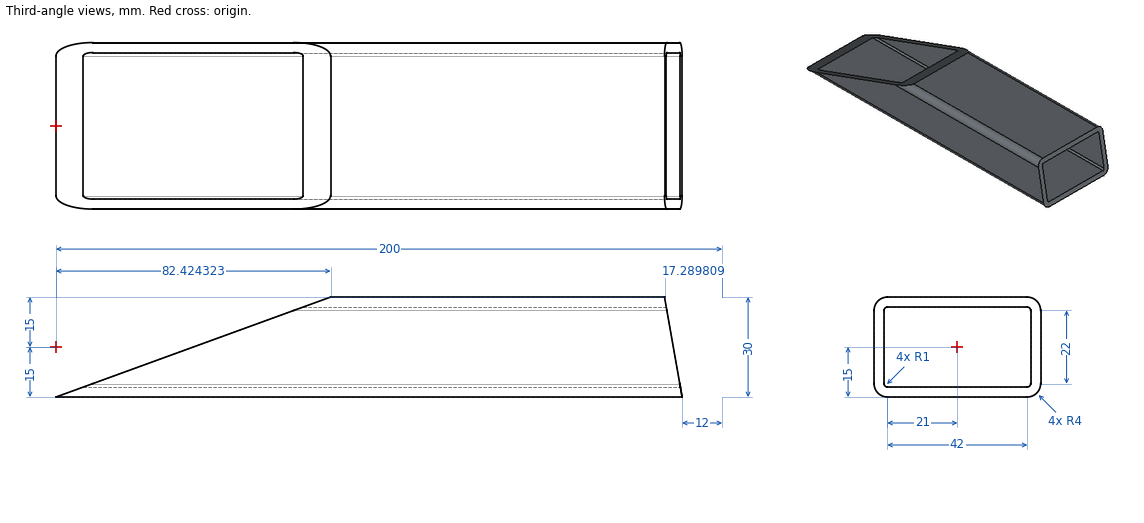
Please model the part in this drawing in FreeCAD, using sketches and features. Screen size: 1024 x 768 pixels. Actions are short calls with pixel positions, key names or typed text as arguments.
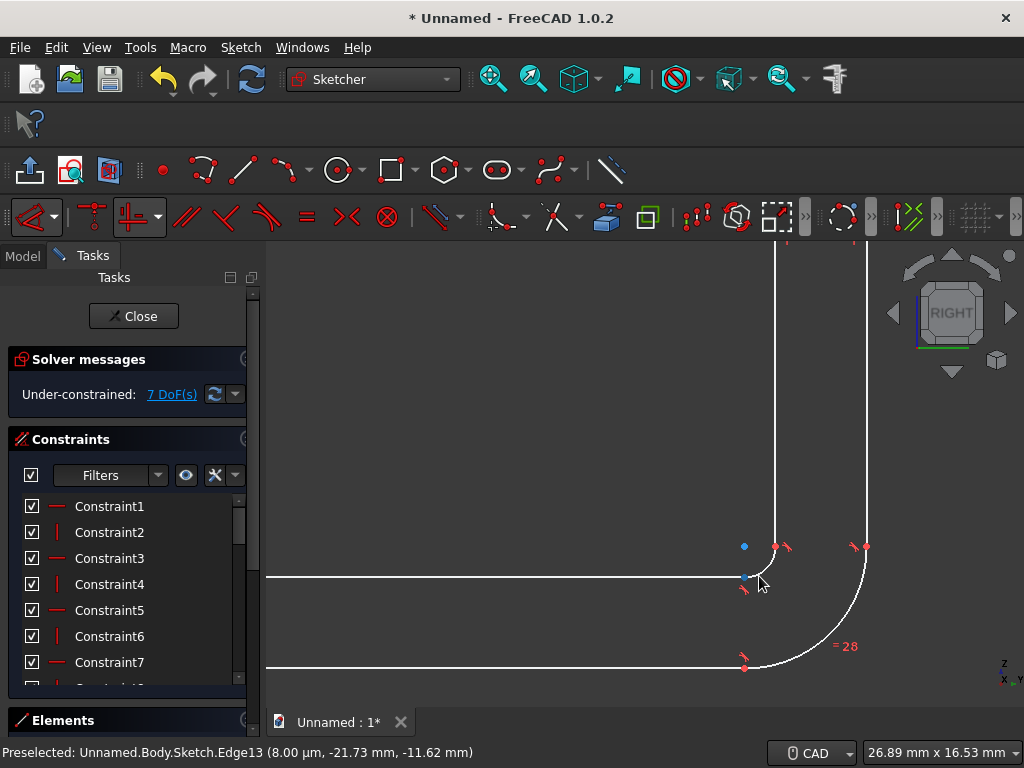
click(759, 574)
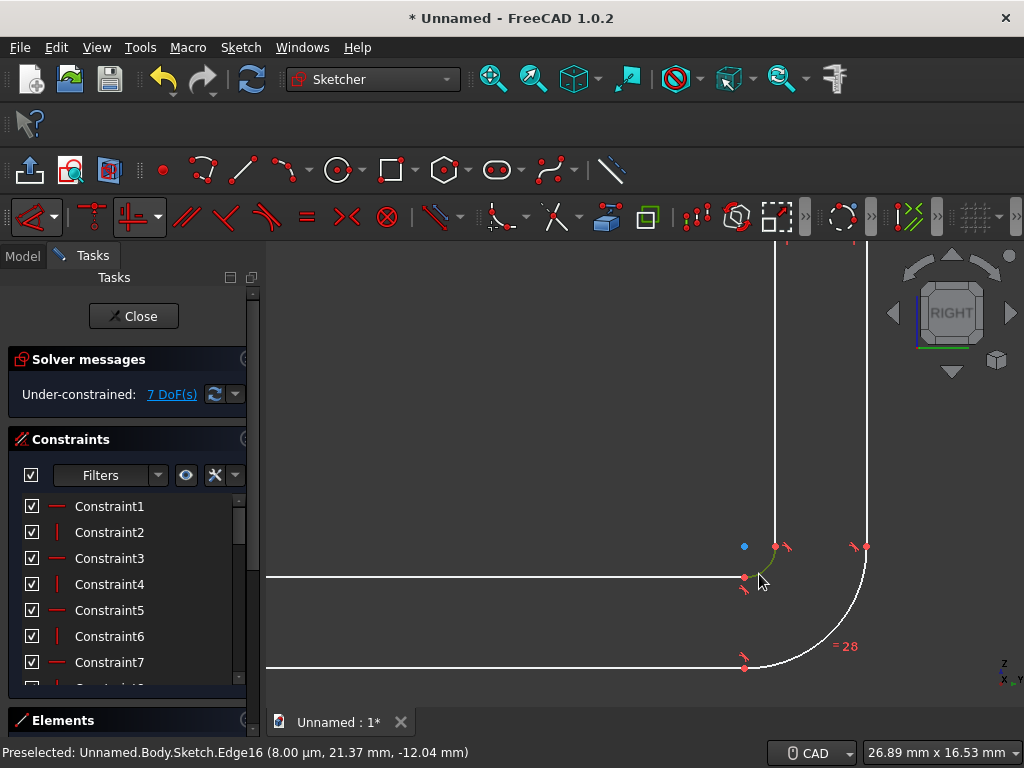
click(308, 218)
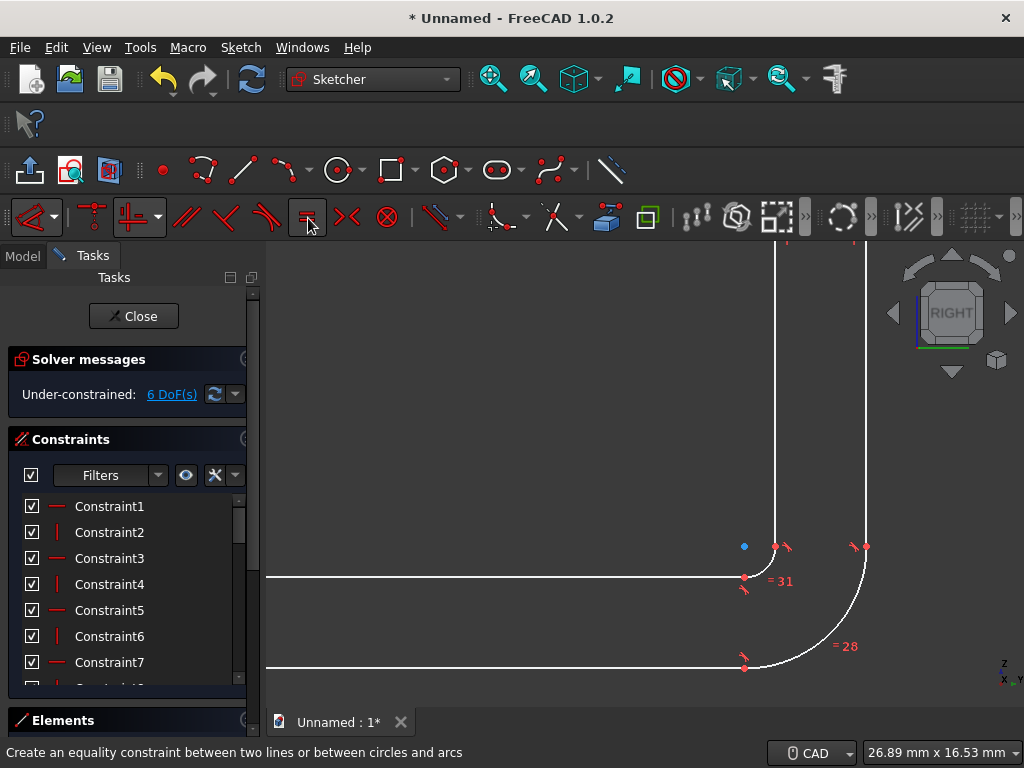
click(30, 218)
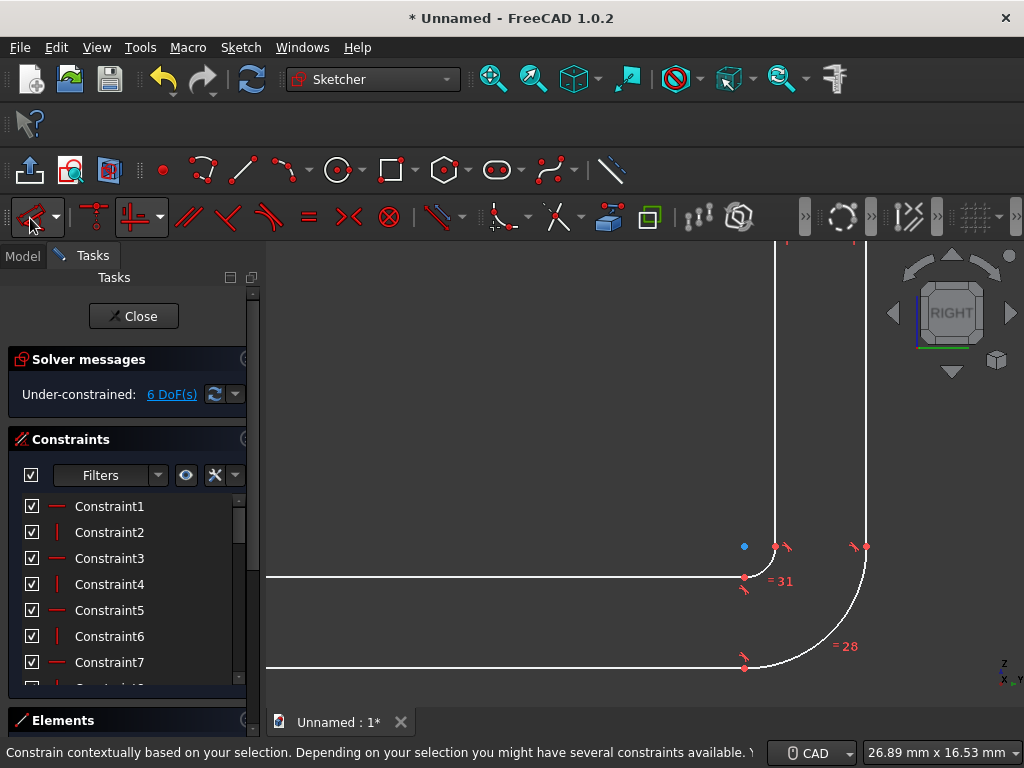
click(800, 655)
click(608, 617)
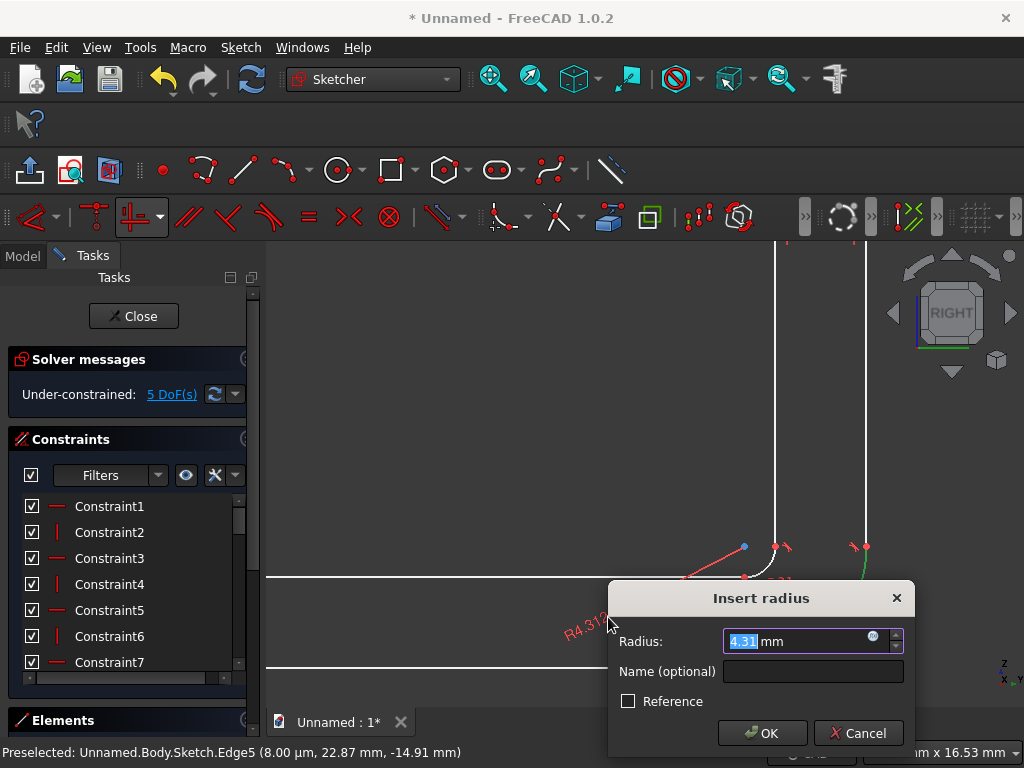
text(4)
key(Return)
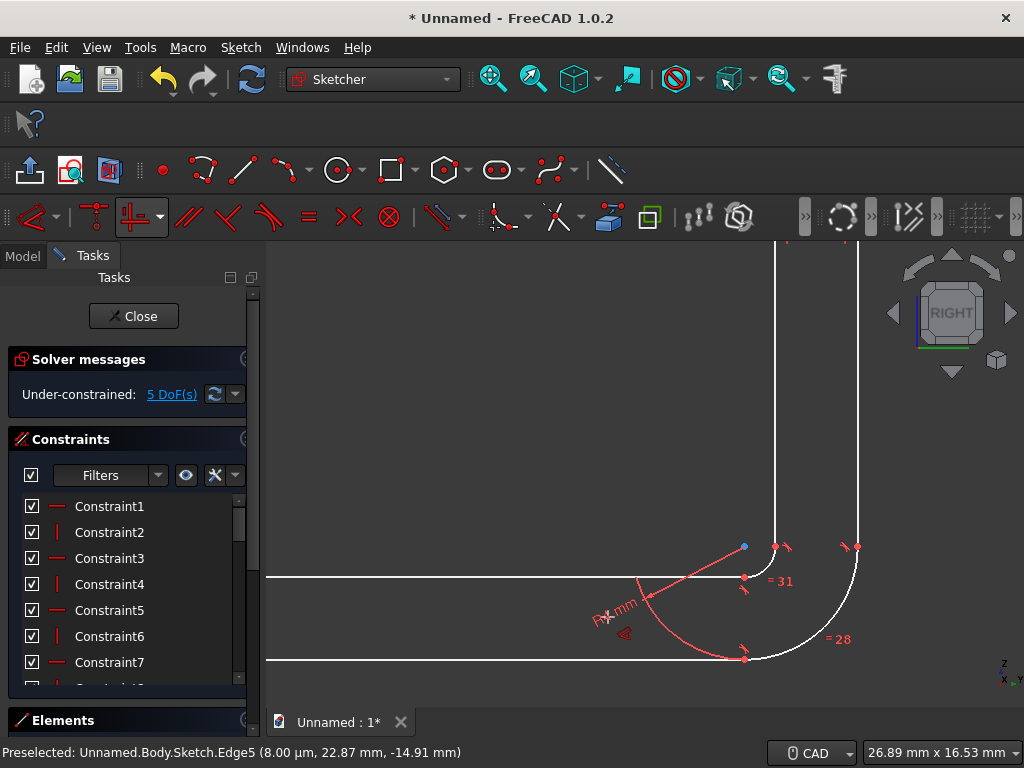
scroll(759, 576, down, 6)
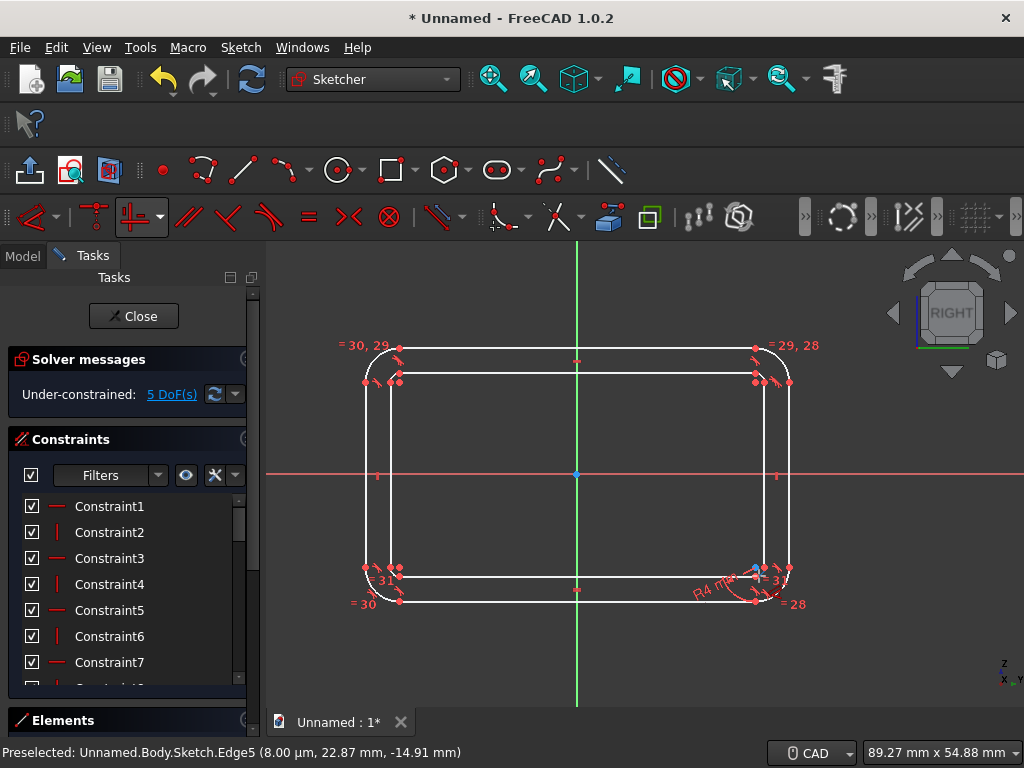
scroll(392, 572, up, 8)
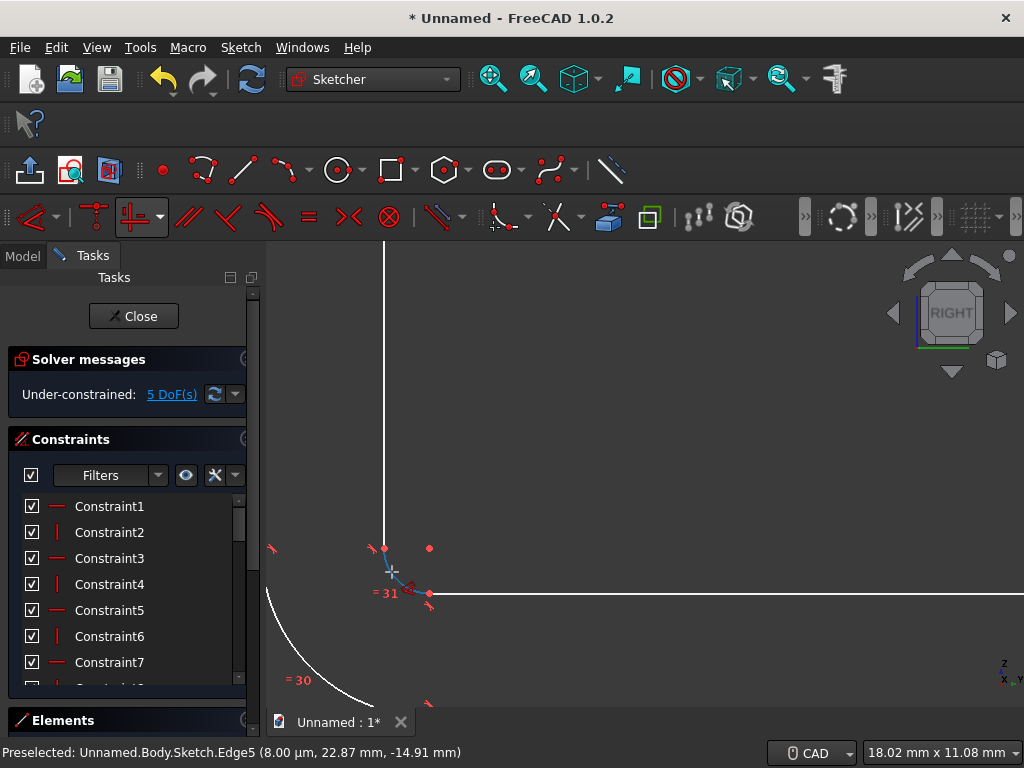
click(389, 569)
click(361, 584)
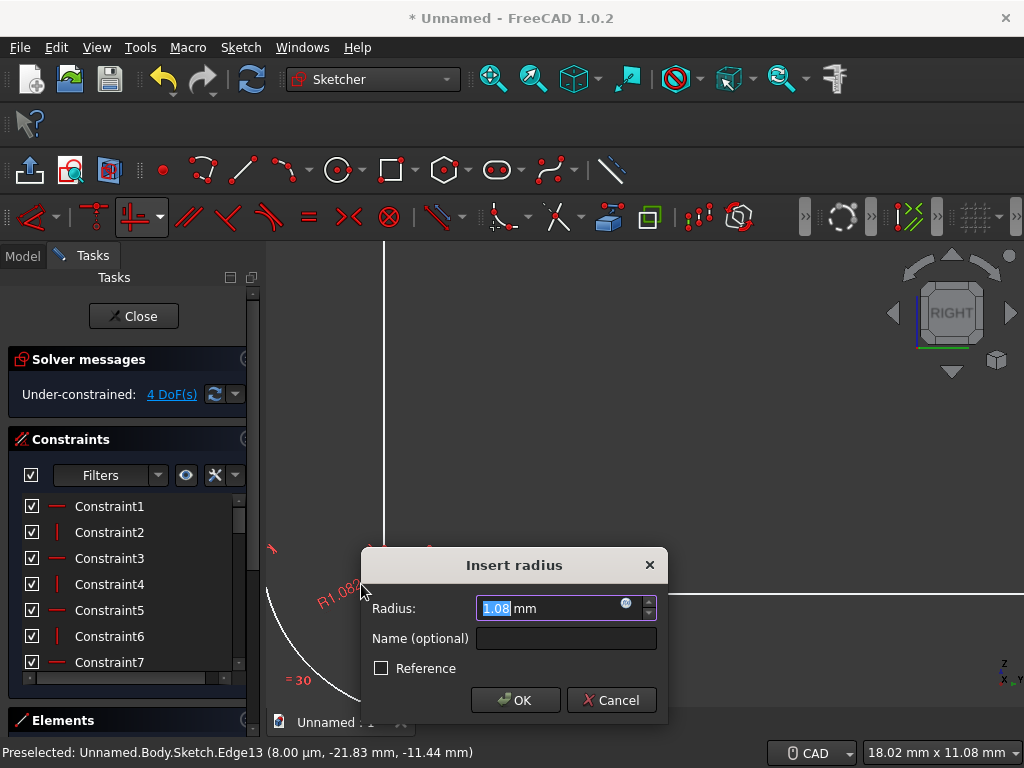
text(1)
key(Return)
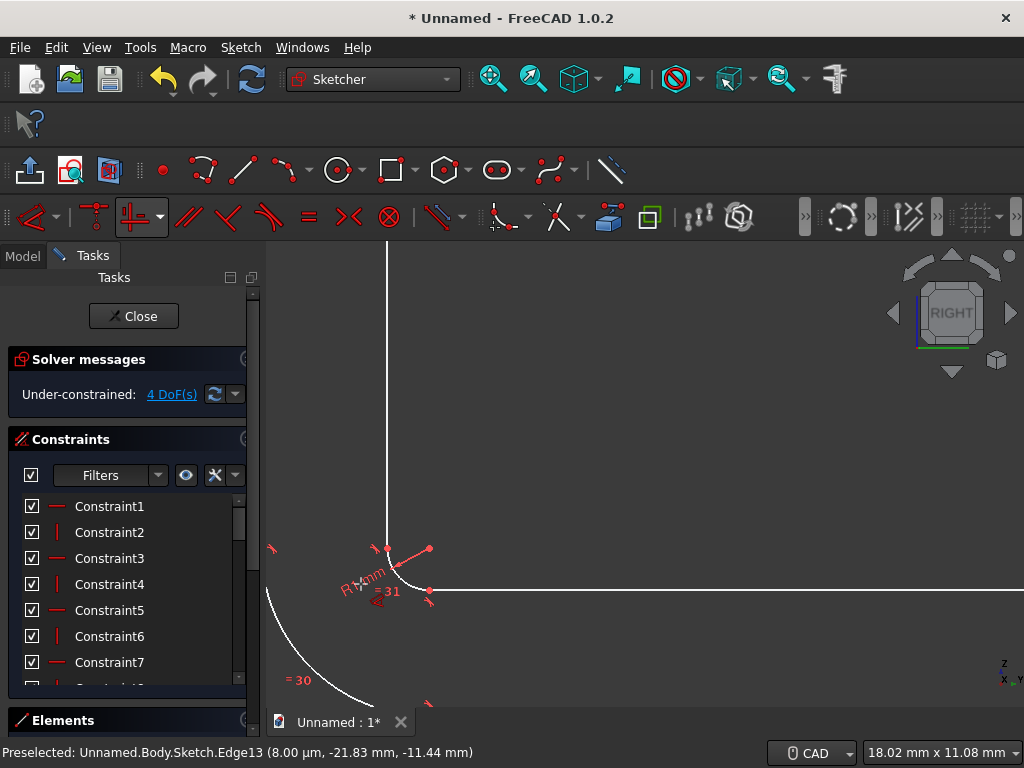
scroll(392, 572, down, 8)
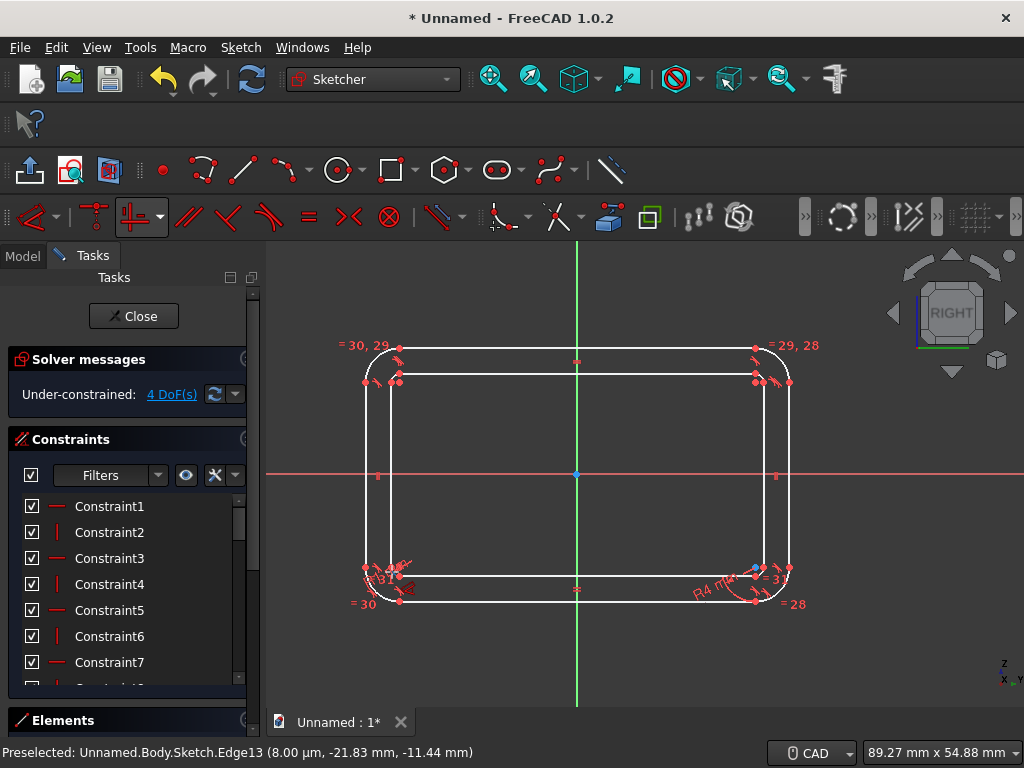
click(506, 602)
click(496, 636)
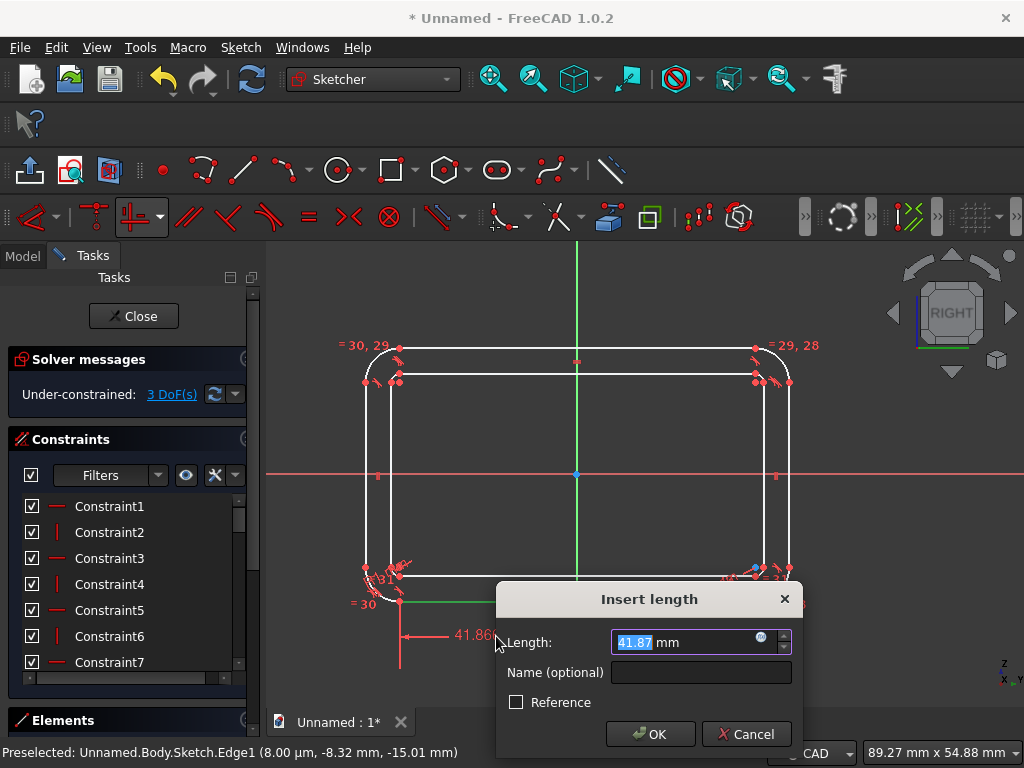
text(42)
key(Return)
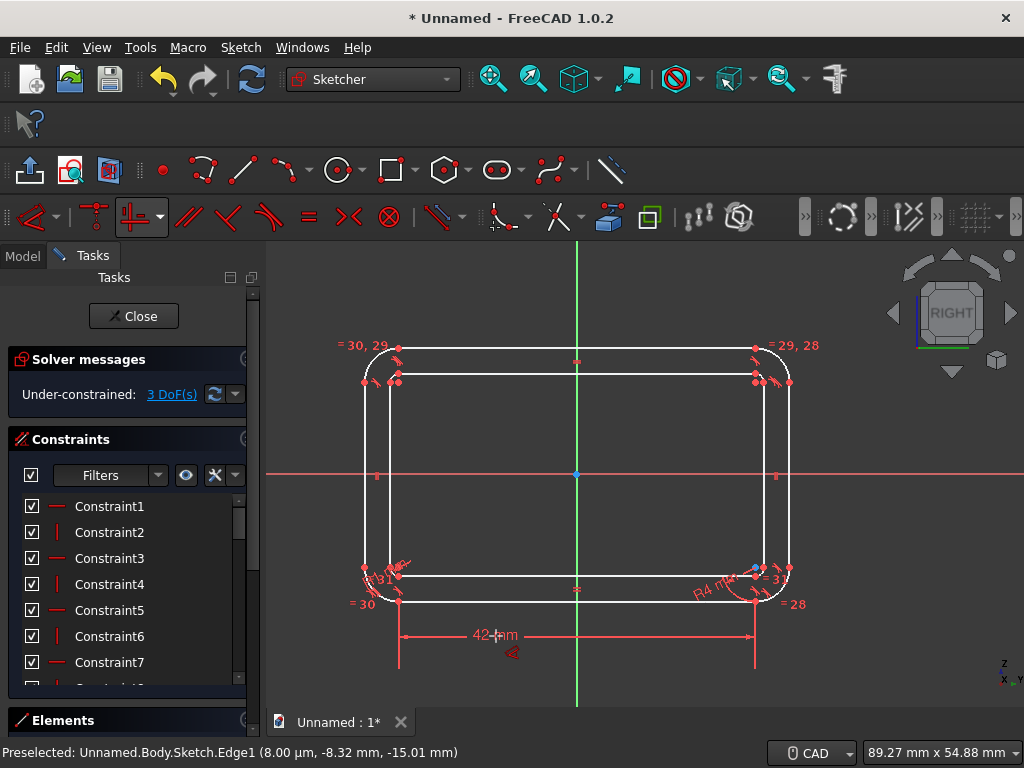
click(789, 512)
click(823, 432)